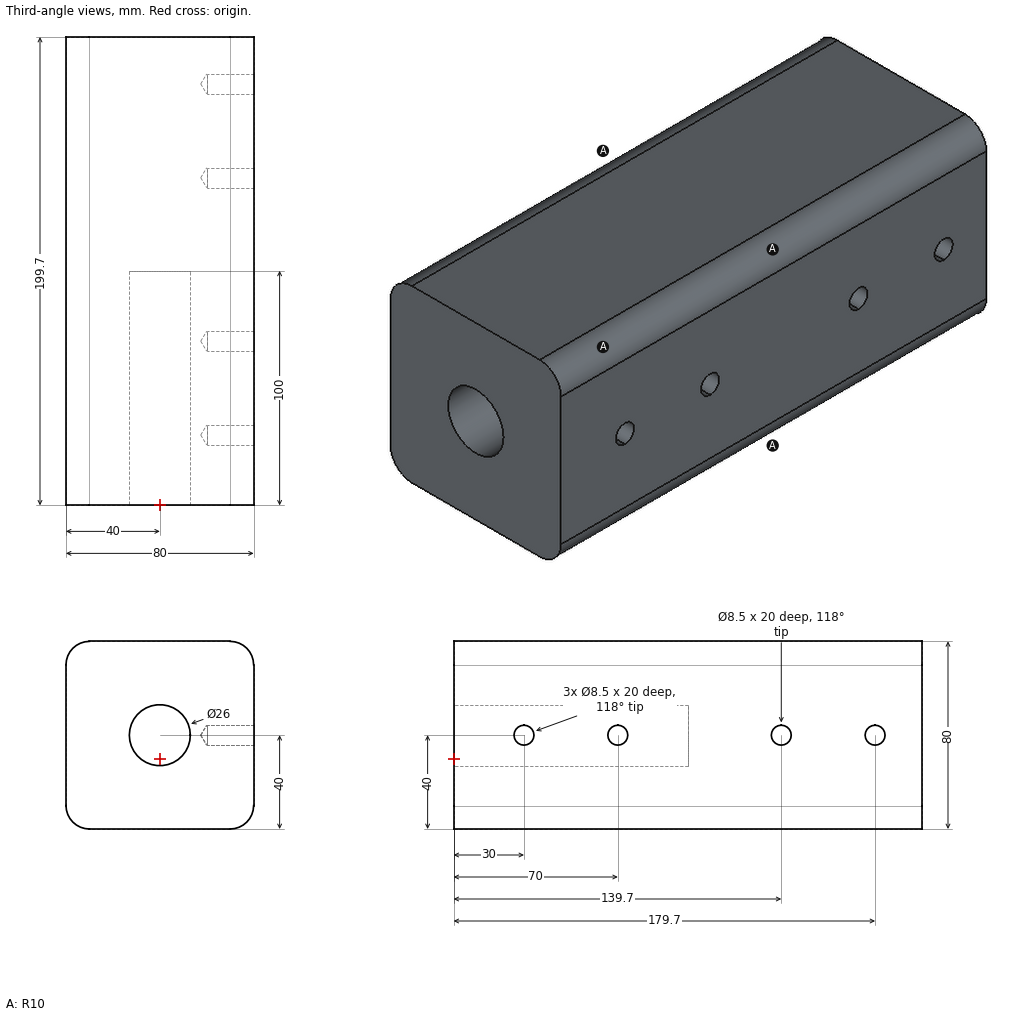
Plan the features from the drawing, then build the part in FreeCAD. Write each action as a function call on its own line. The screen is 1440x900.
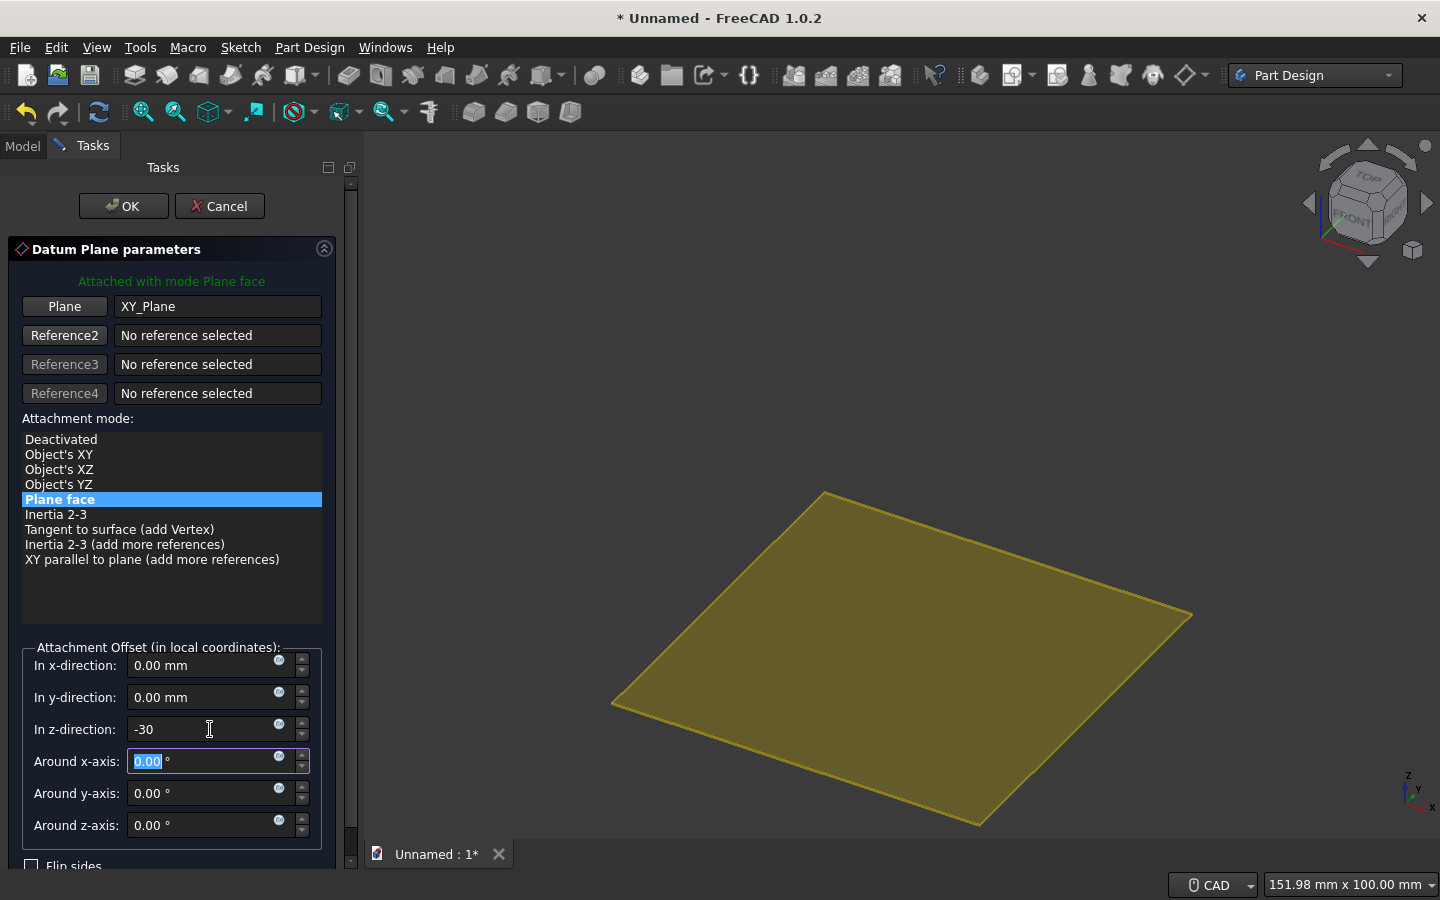
click(124, 206)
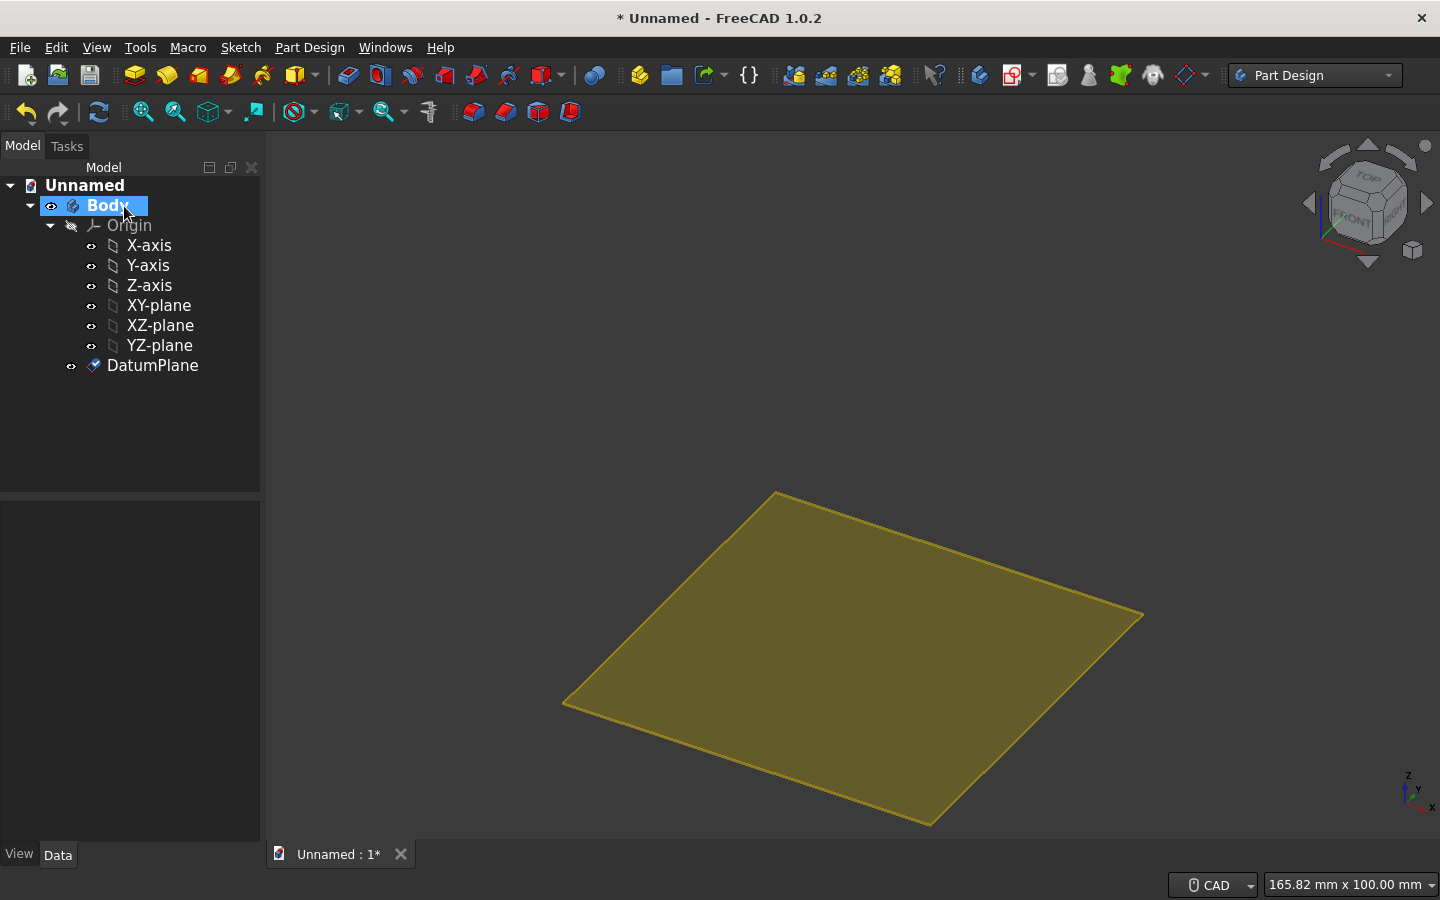
click(116, 366)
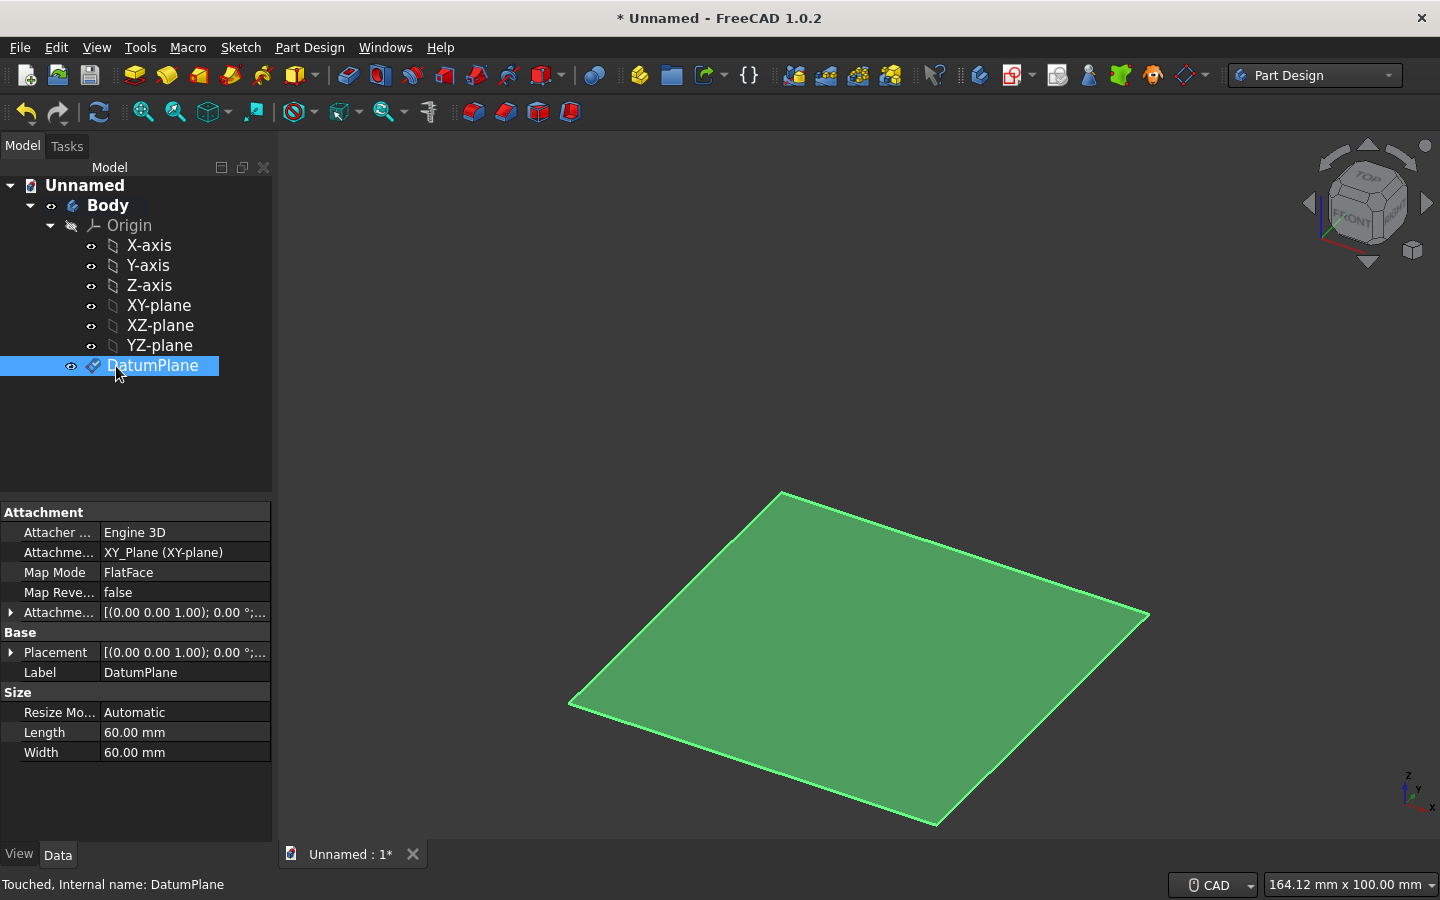
click(1012, 76)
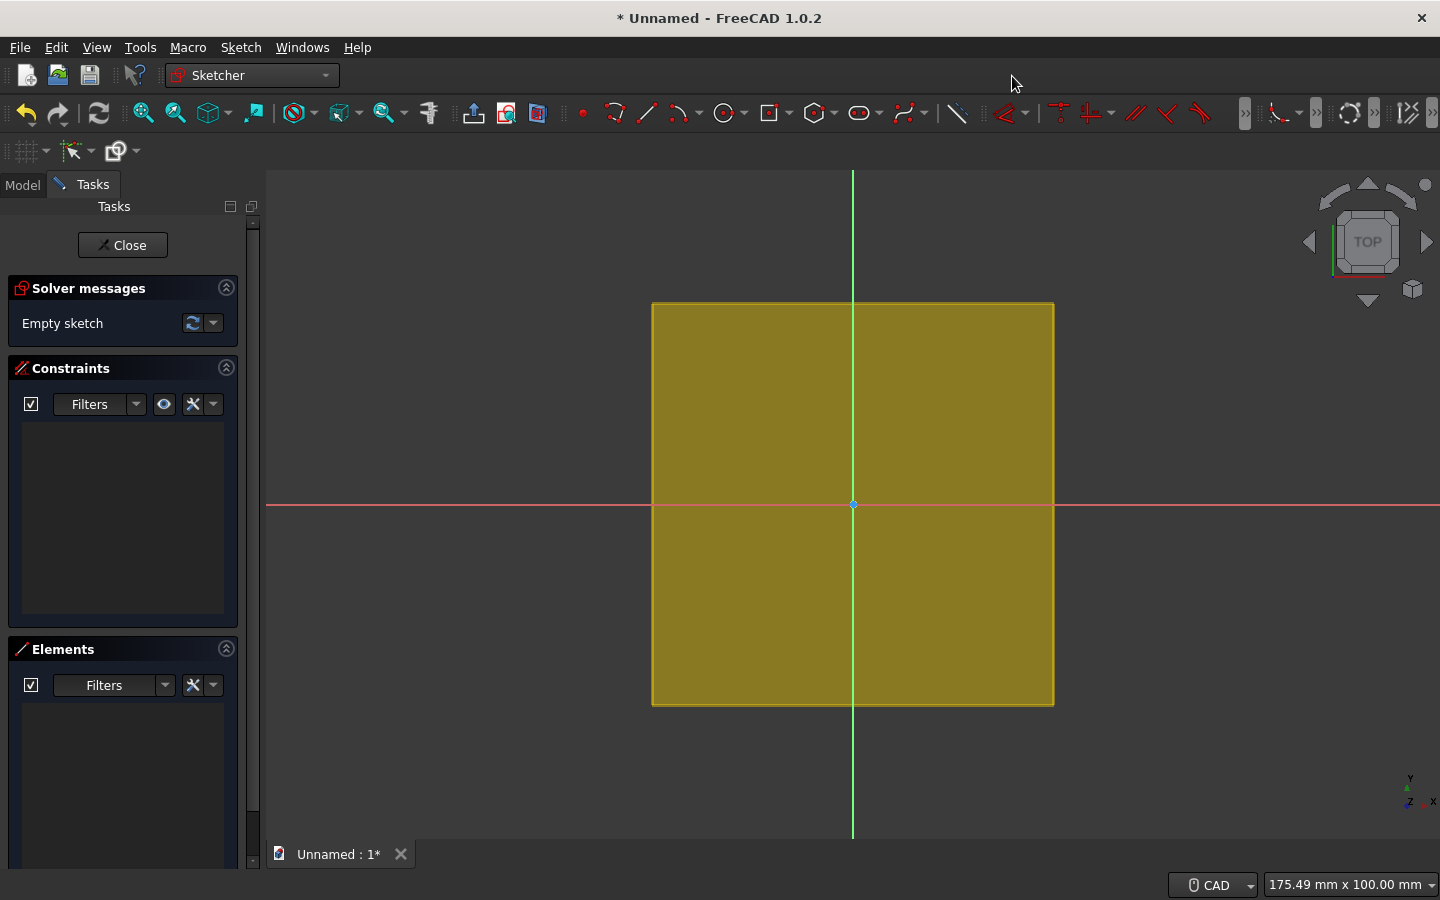
scroll(755, 792, down, 6)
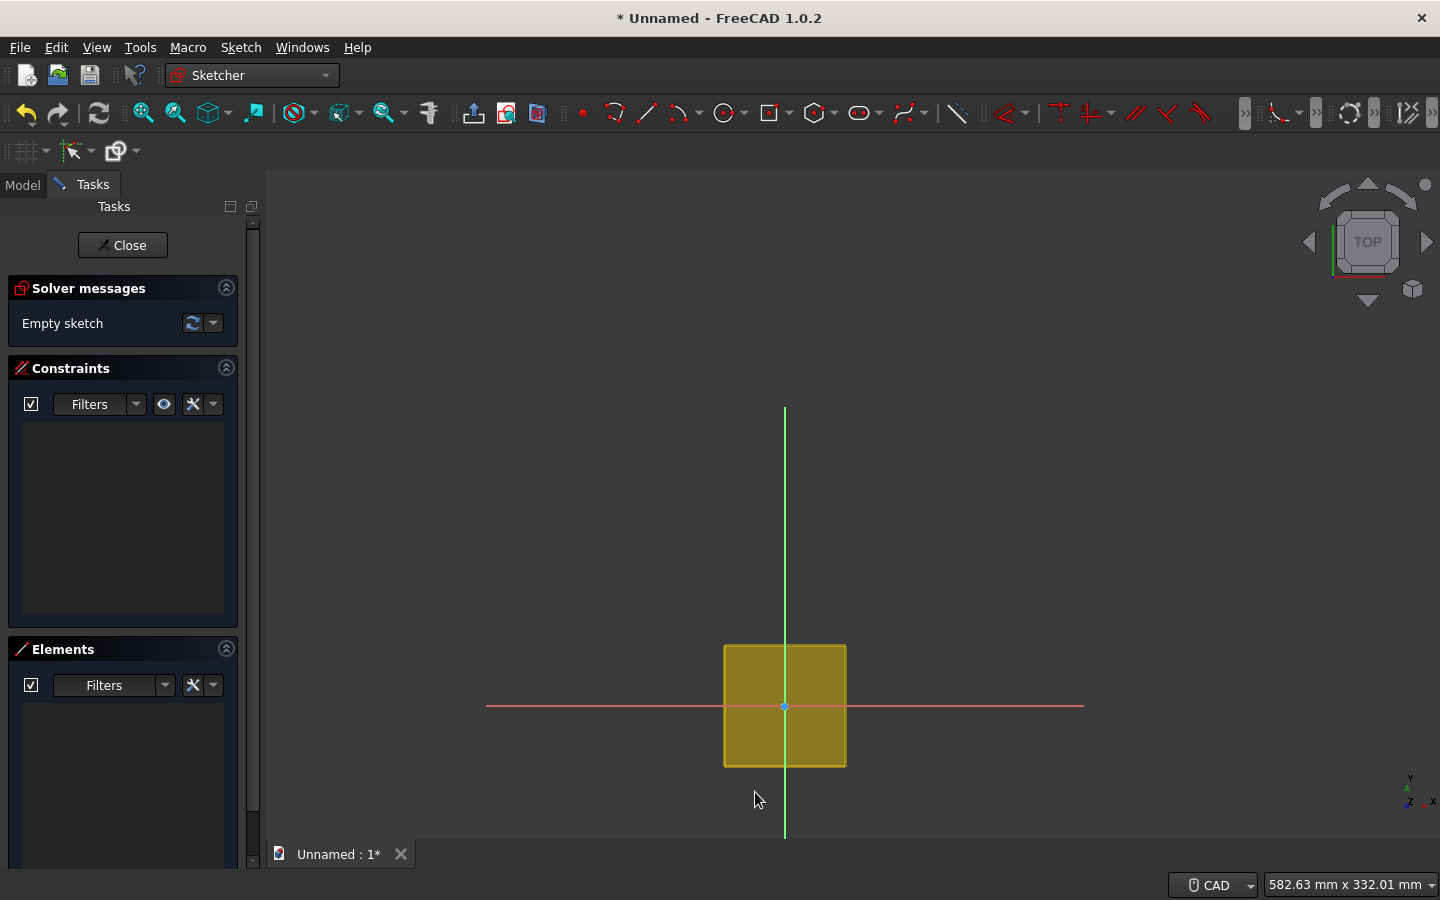
key(g)
key(r)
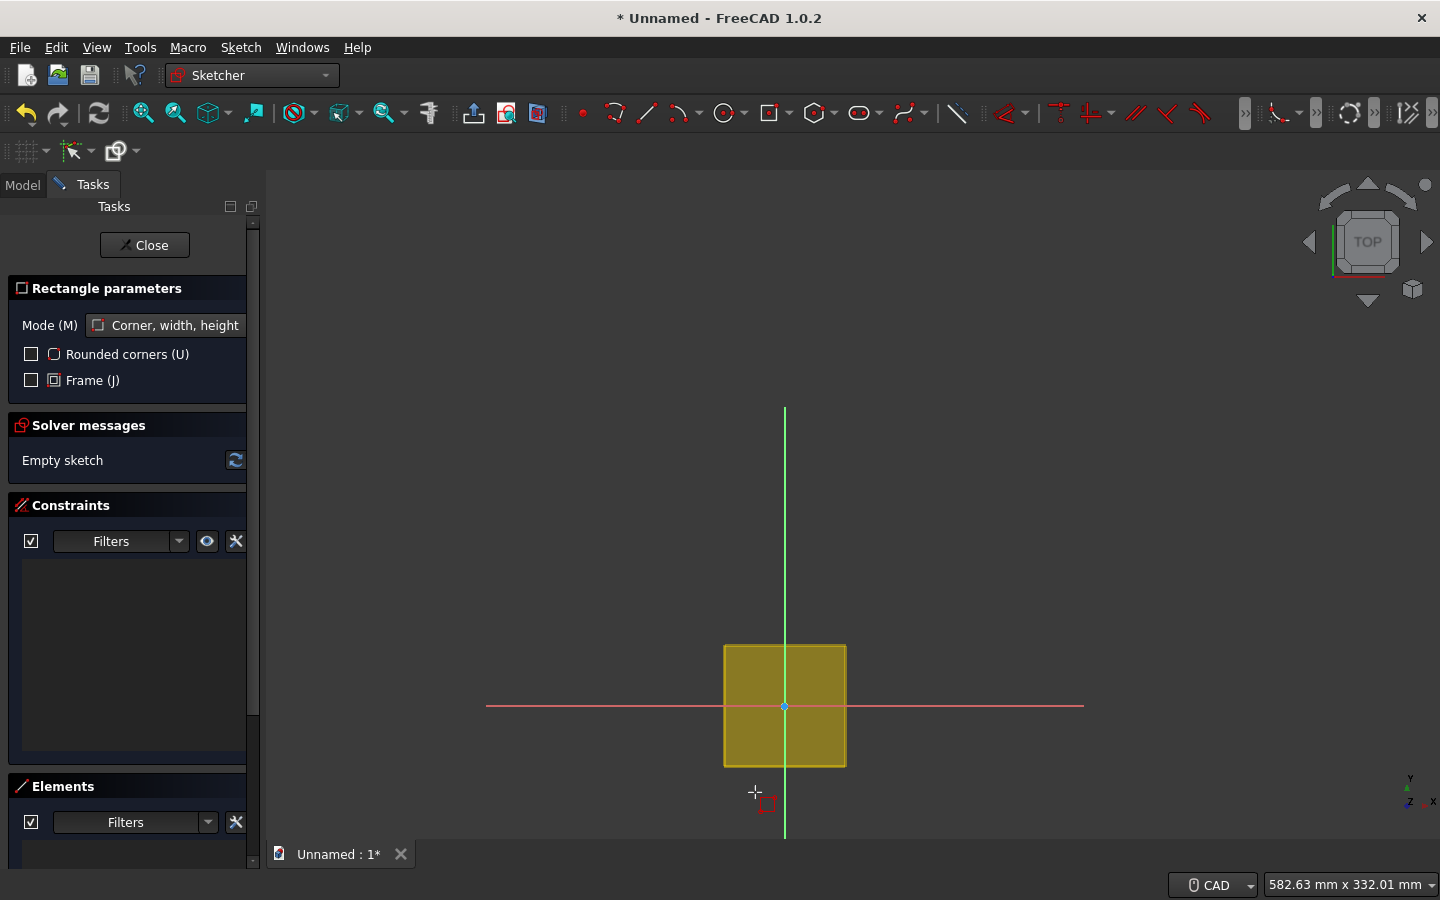
click(704, 304)
click(865, 706)
key(Escape)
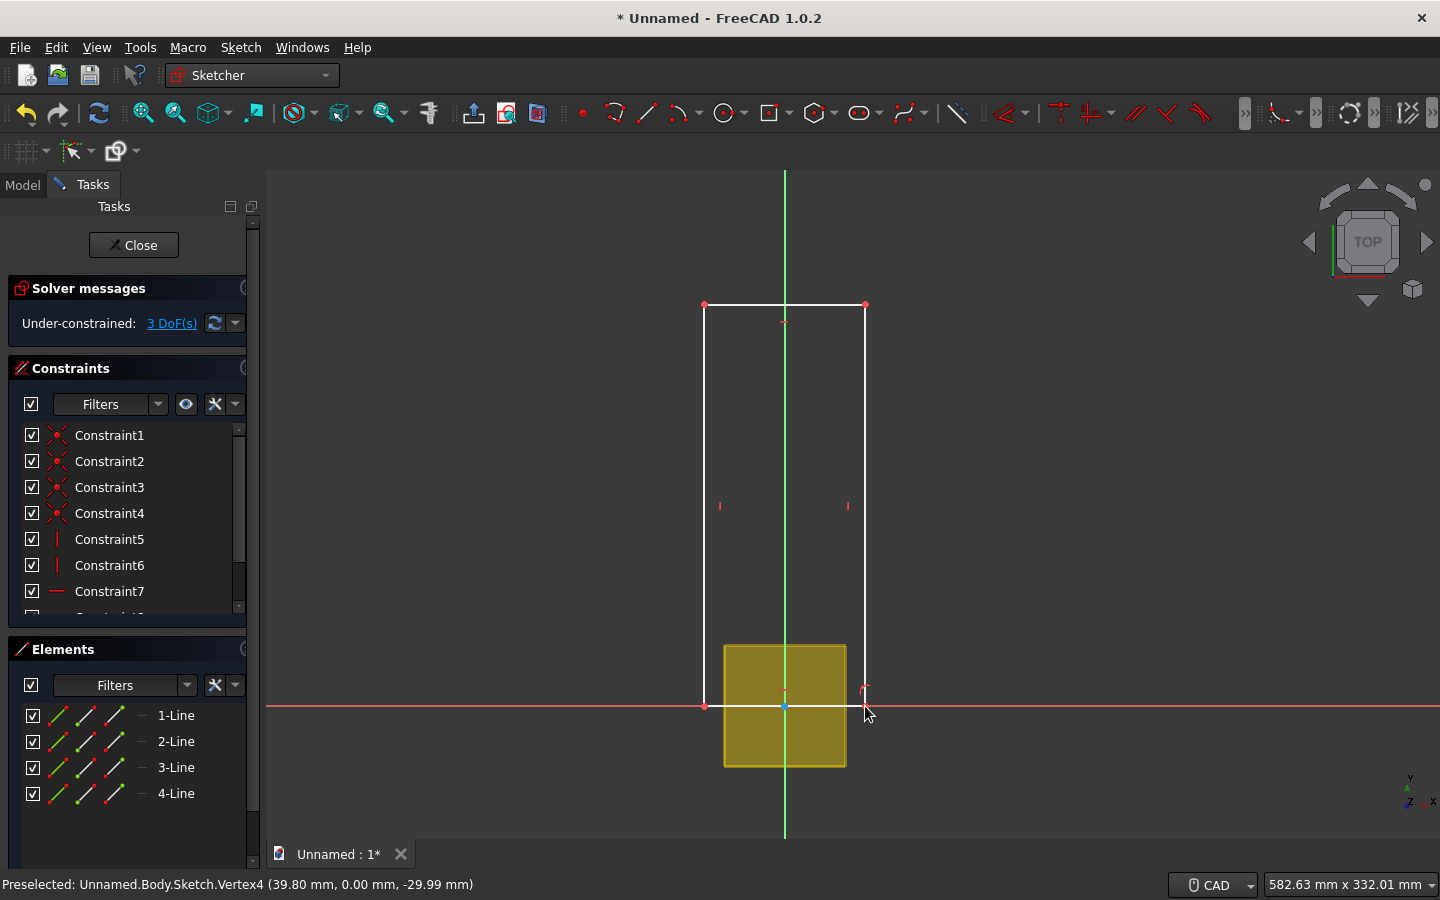
click(752, 706)